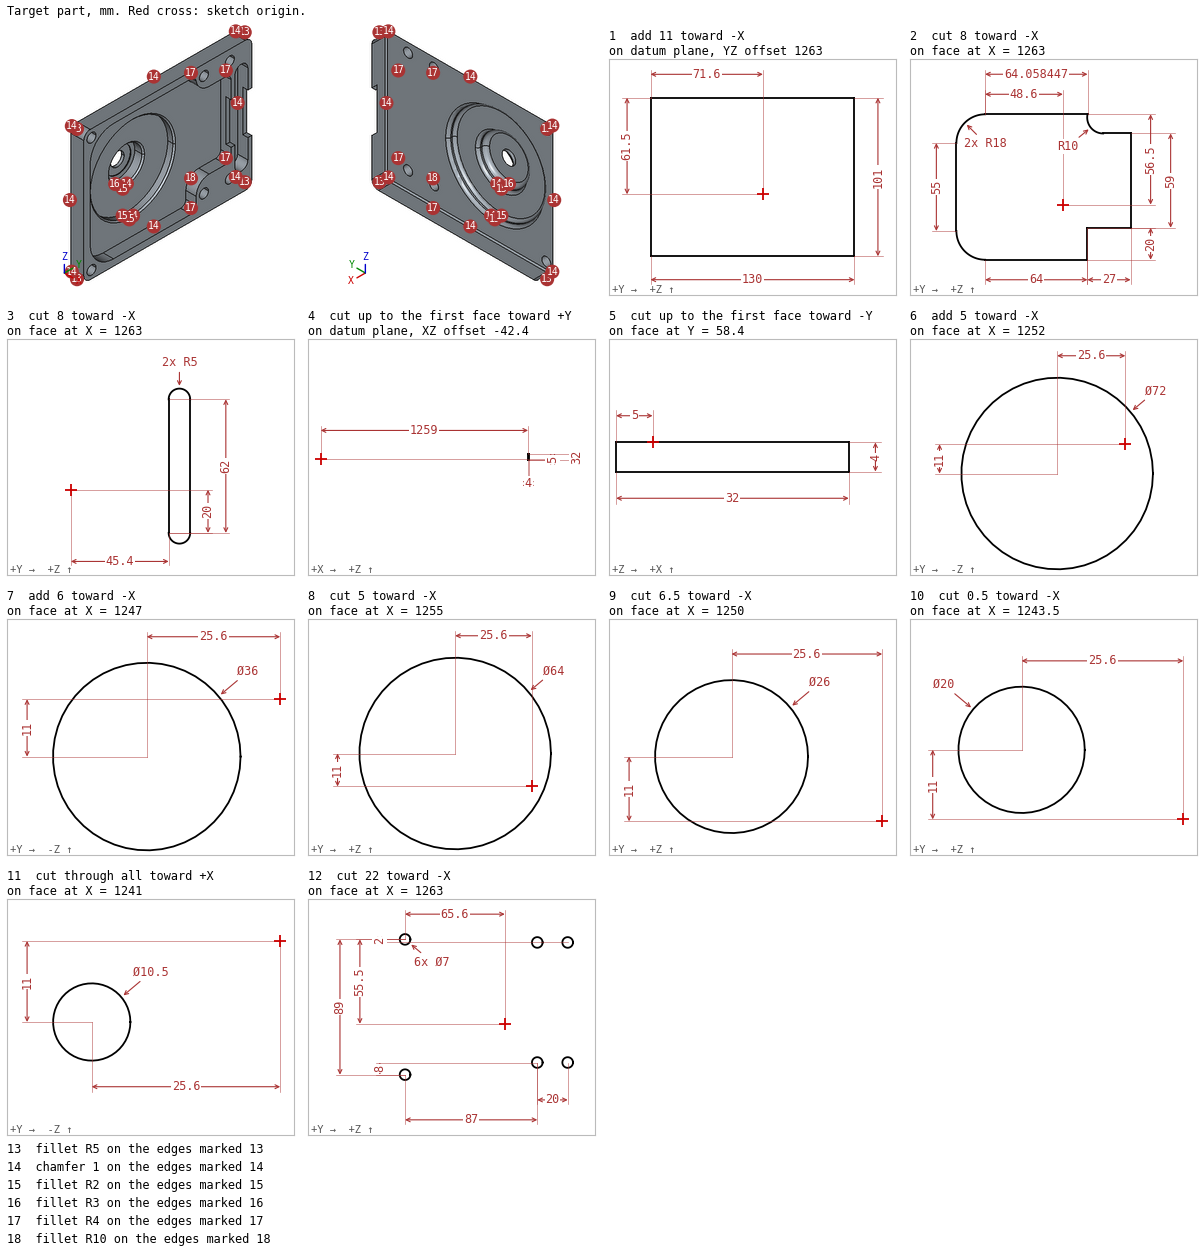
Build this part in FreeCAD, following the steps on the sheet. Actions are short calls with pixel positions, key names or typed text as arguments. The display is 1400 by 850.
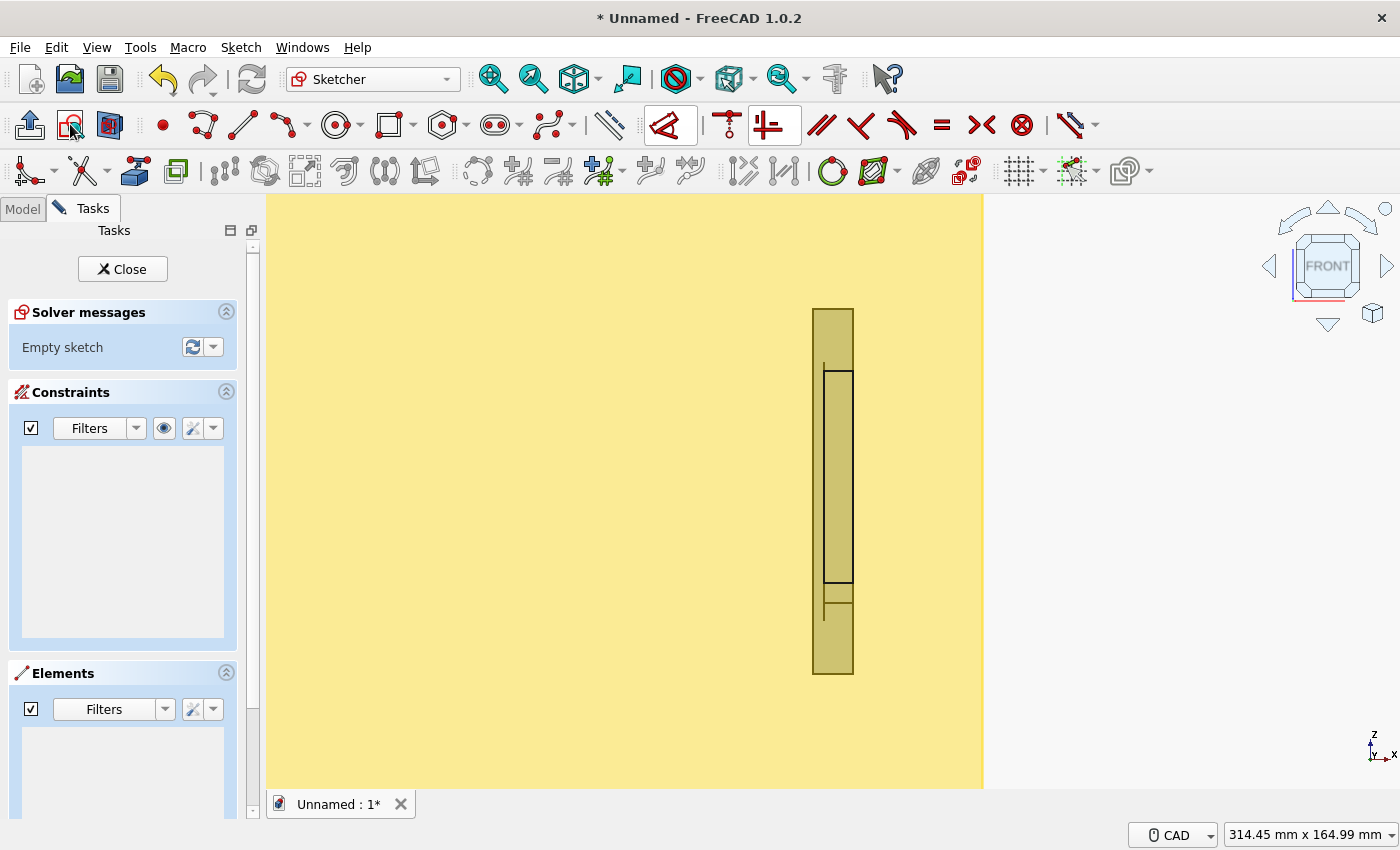
scroll(881, 492, up, 6)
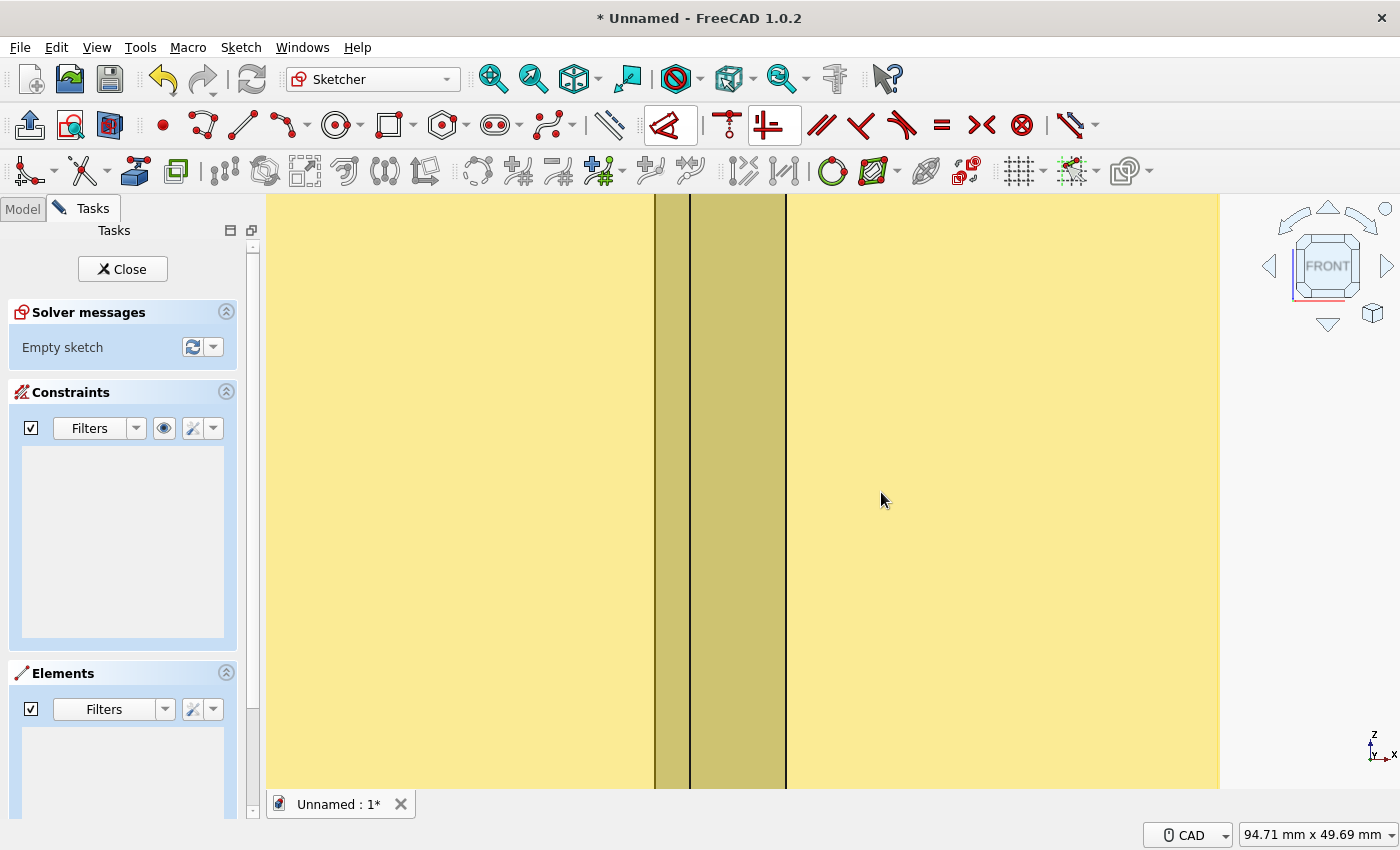
key(g)
key(r)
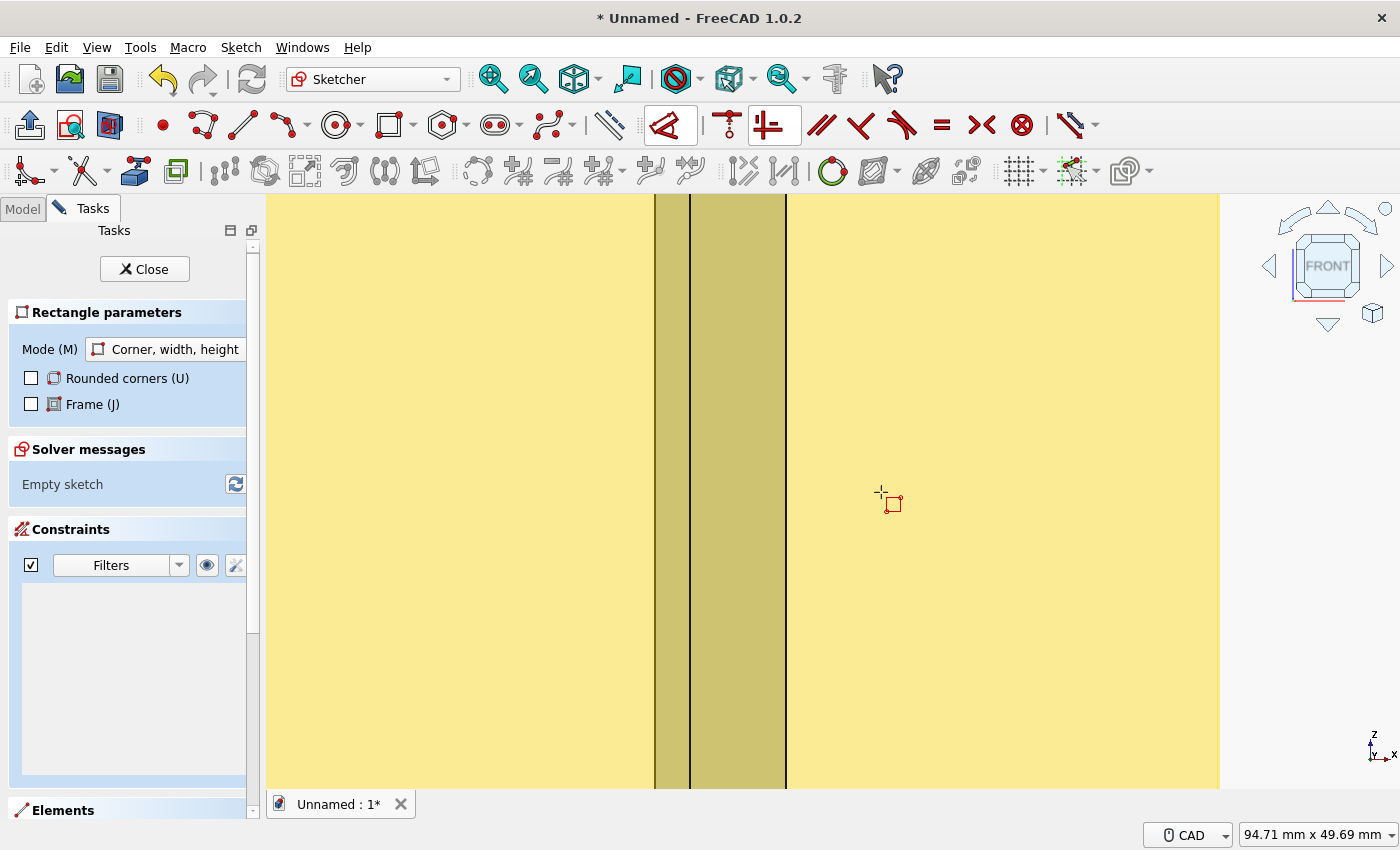
click(738, 298)
move(786, 681)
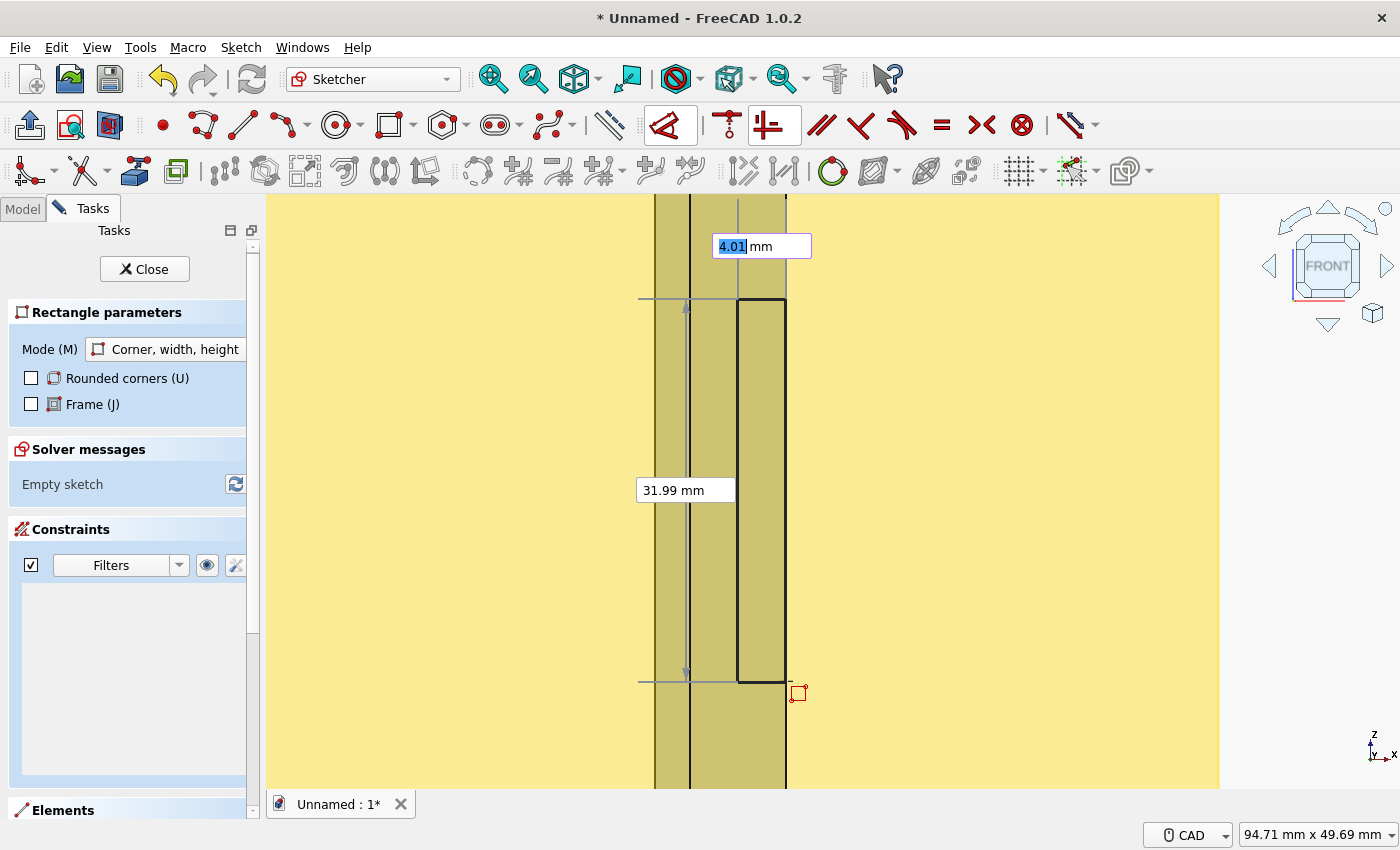
text(4)
key(Tab)
text(32)
key(Return)
key(Escape)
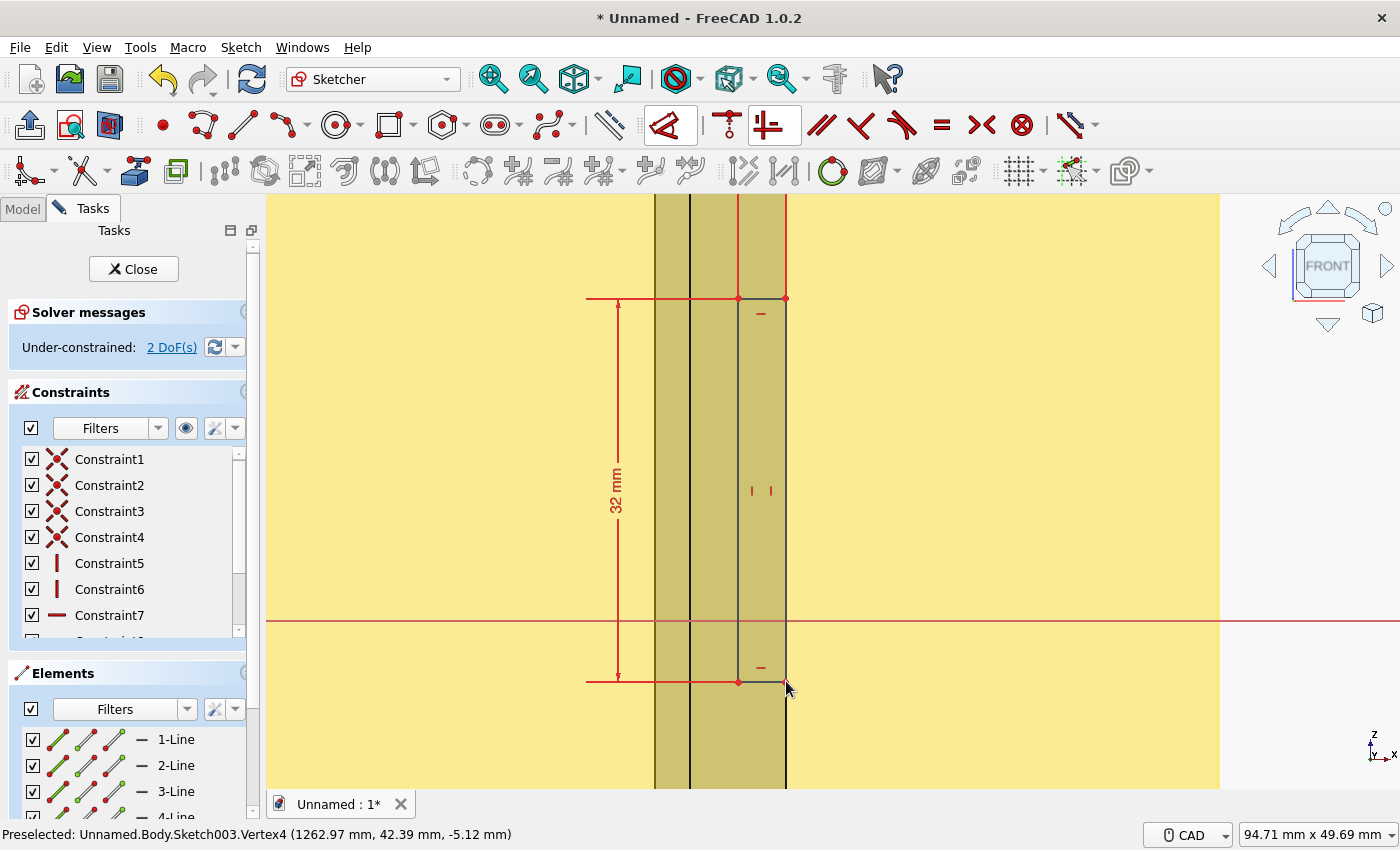
click(738, 682)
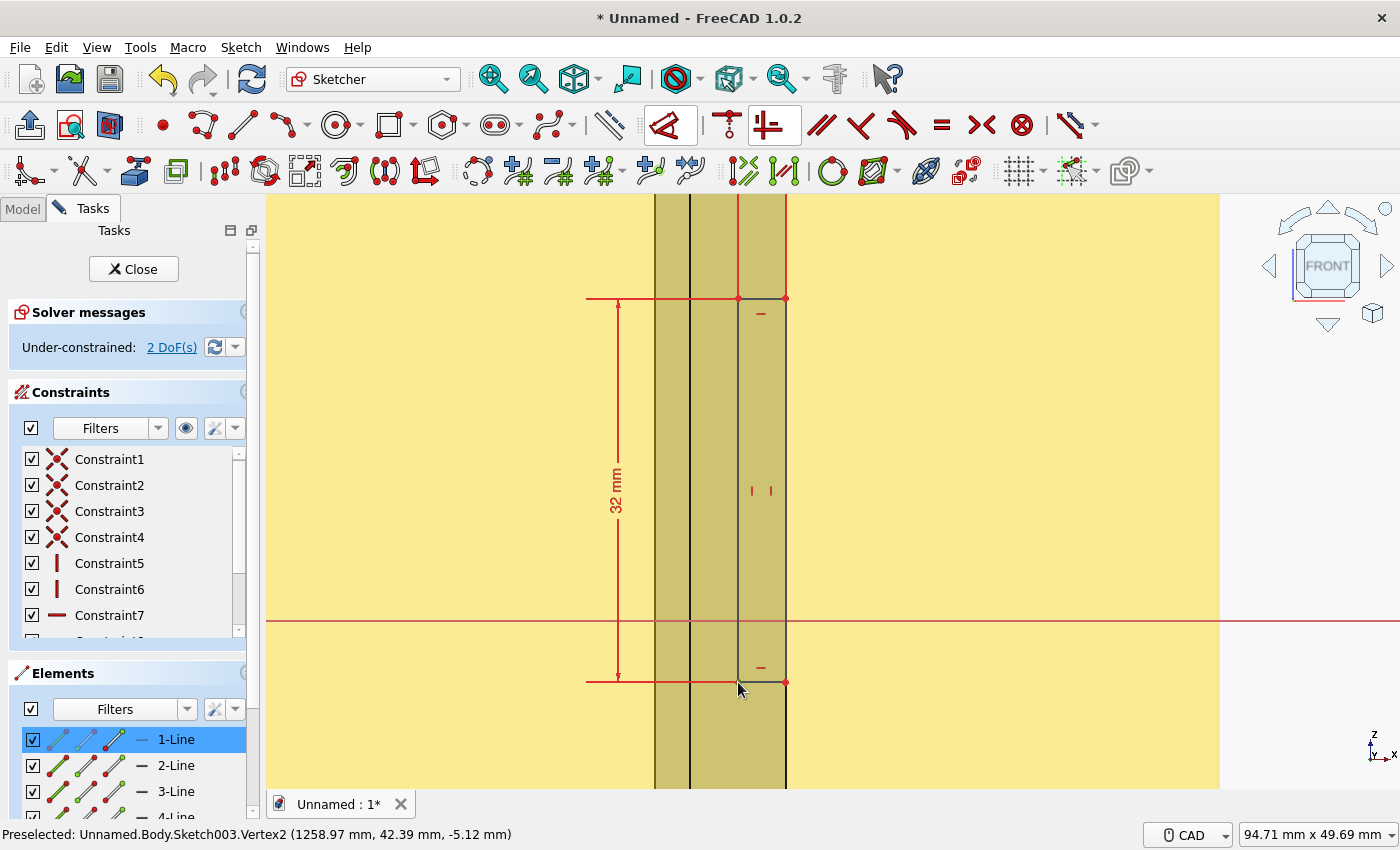
key(i)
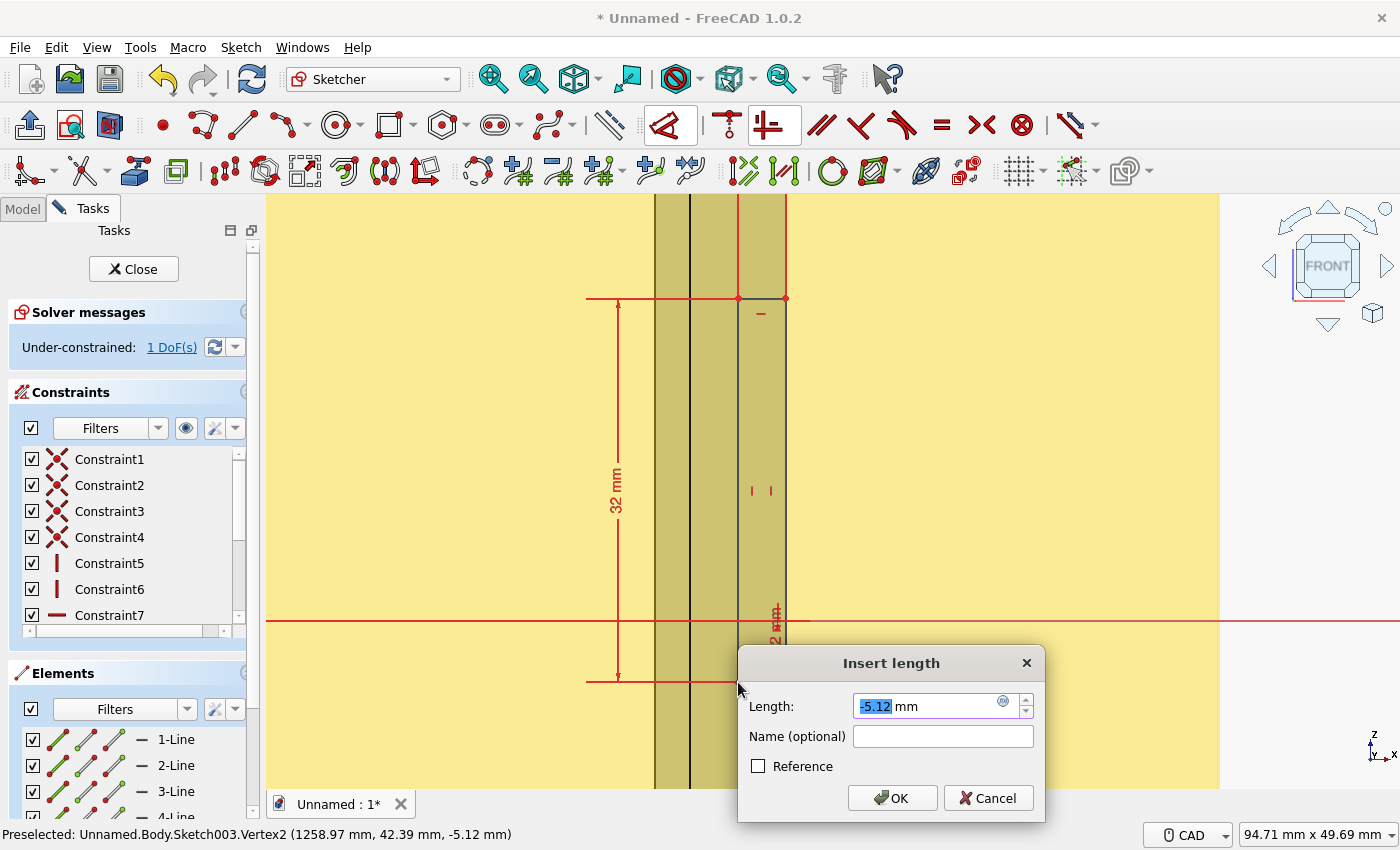
text(-5)
key(Return)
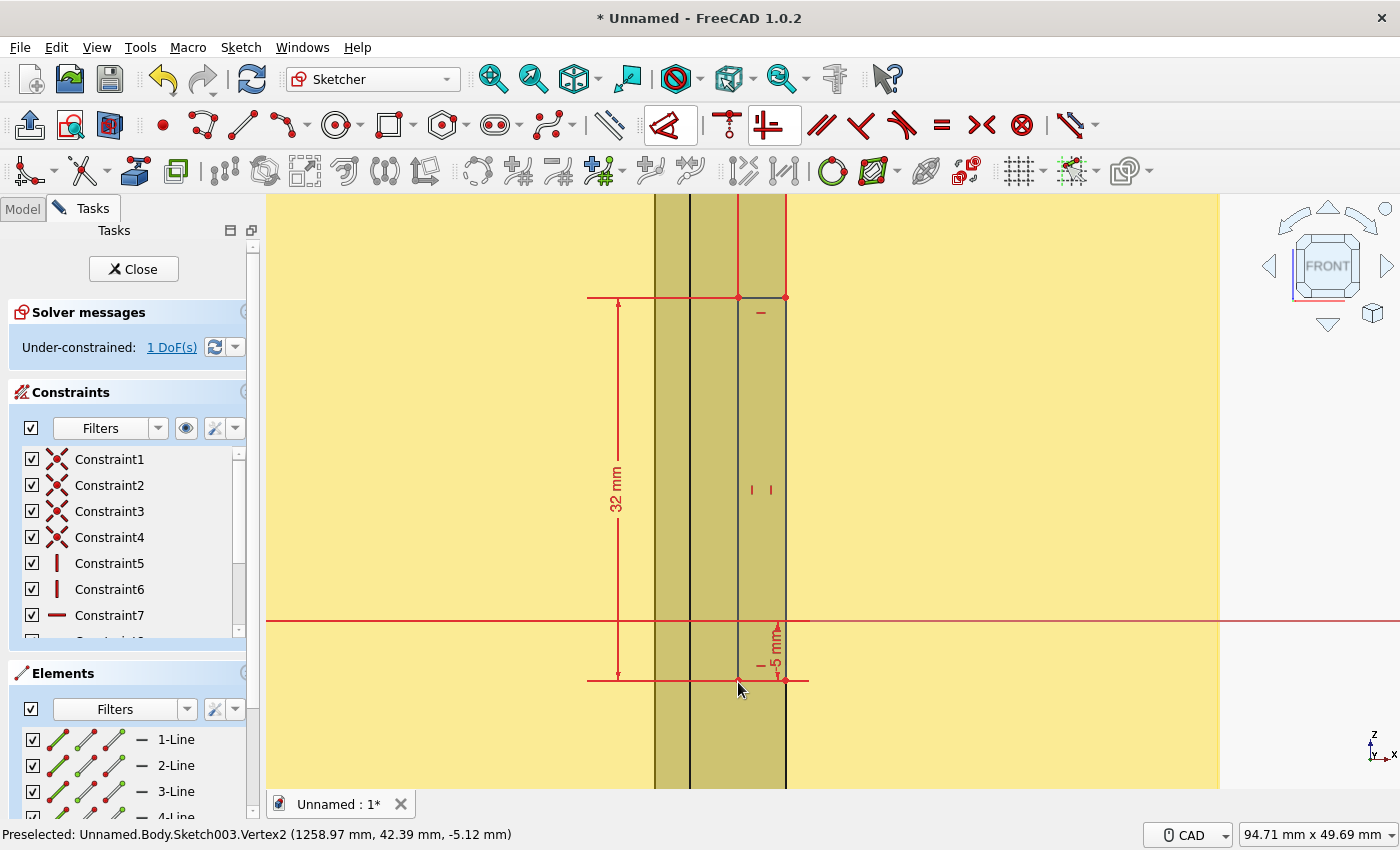
click(738, 298)